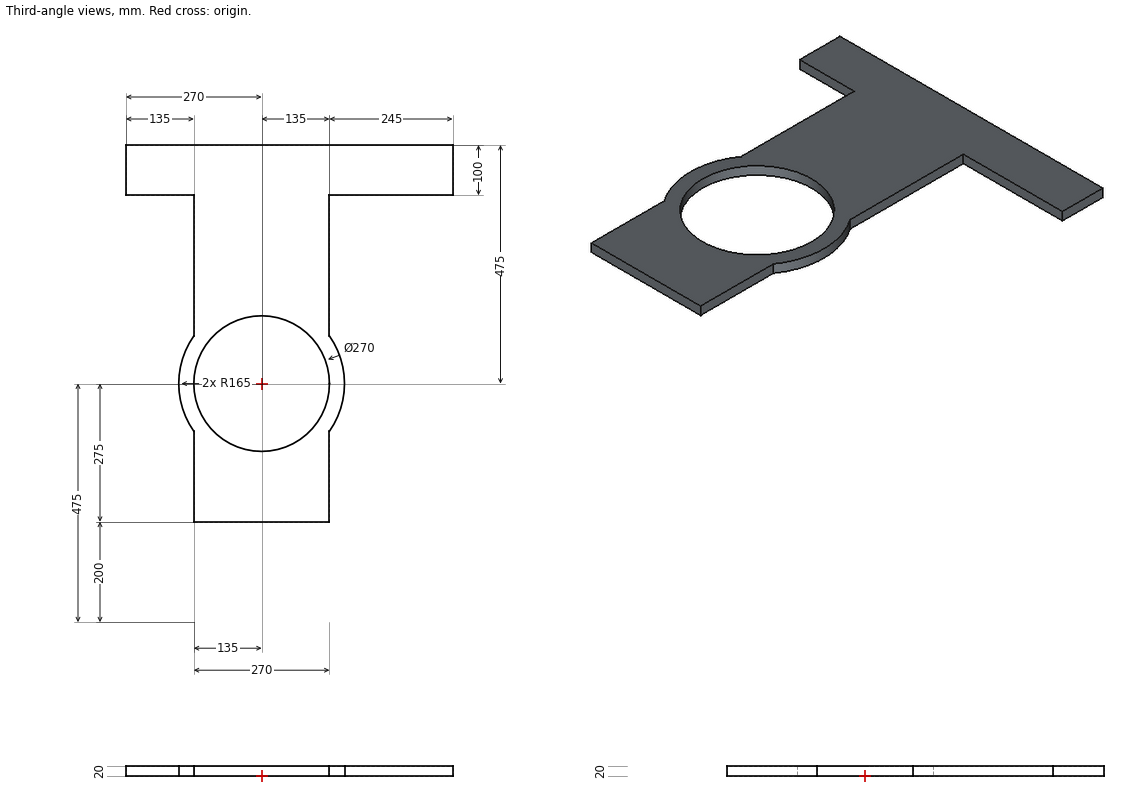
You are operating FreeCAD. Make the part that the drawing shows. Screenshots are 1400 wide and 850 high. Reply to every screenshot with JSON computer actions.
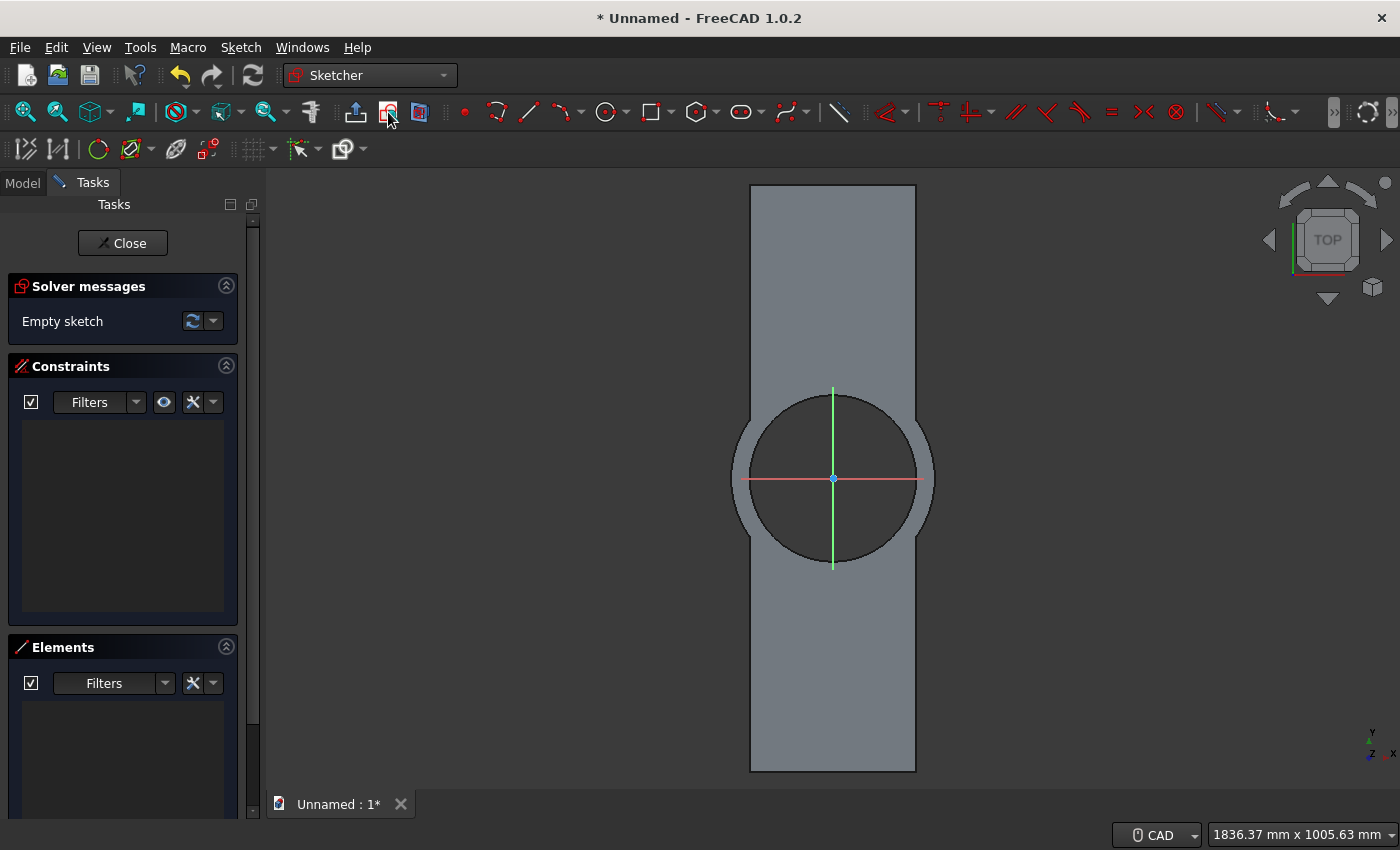
{"action": "scroll", "coordinate": [455, 196], "scroll_direction": "down", "scroll_amount": 1}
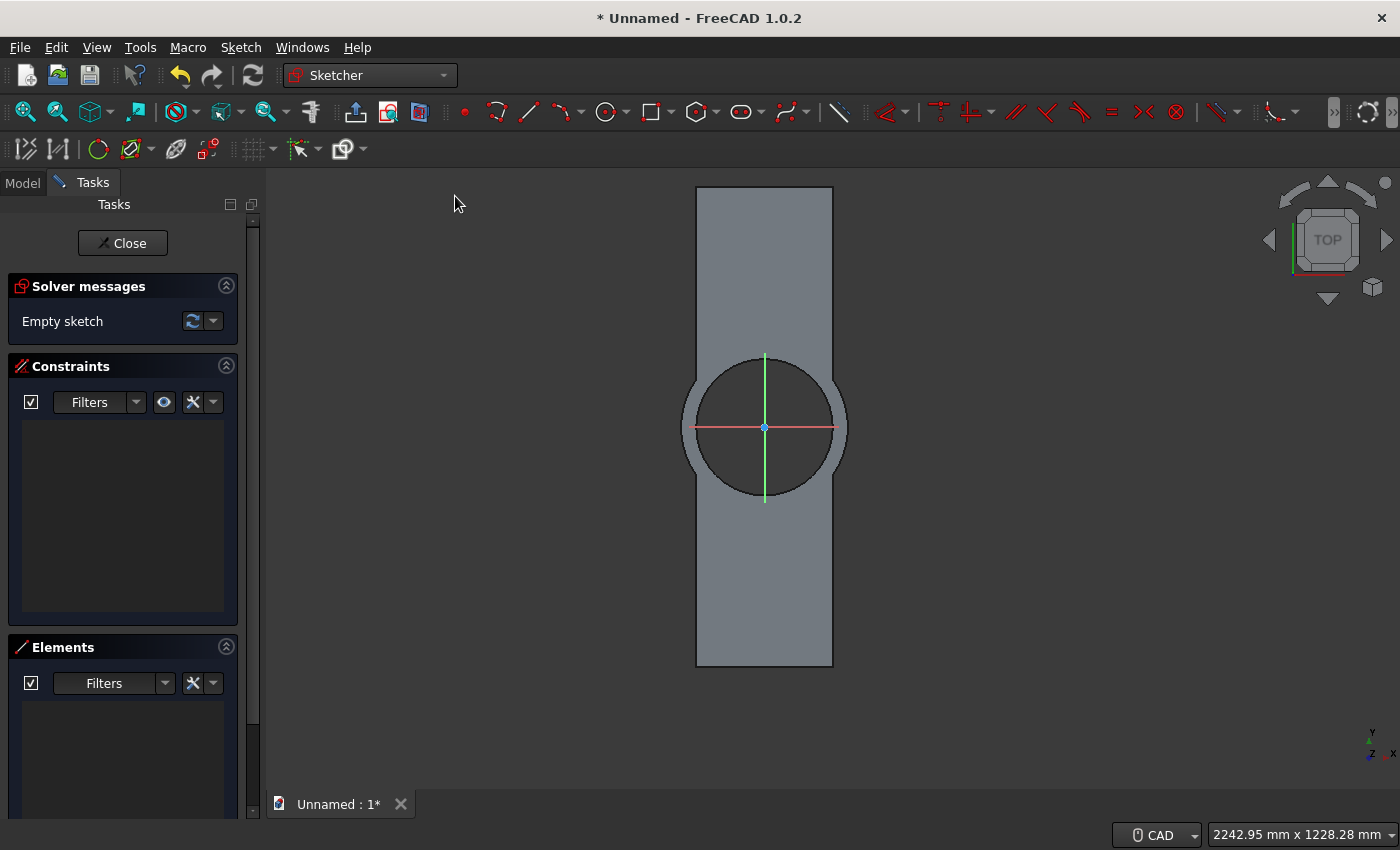
{"action": "scroll", "coordinate": [765, 631], "scroll_direction": "up", "scroll_amount": 3}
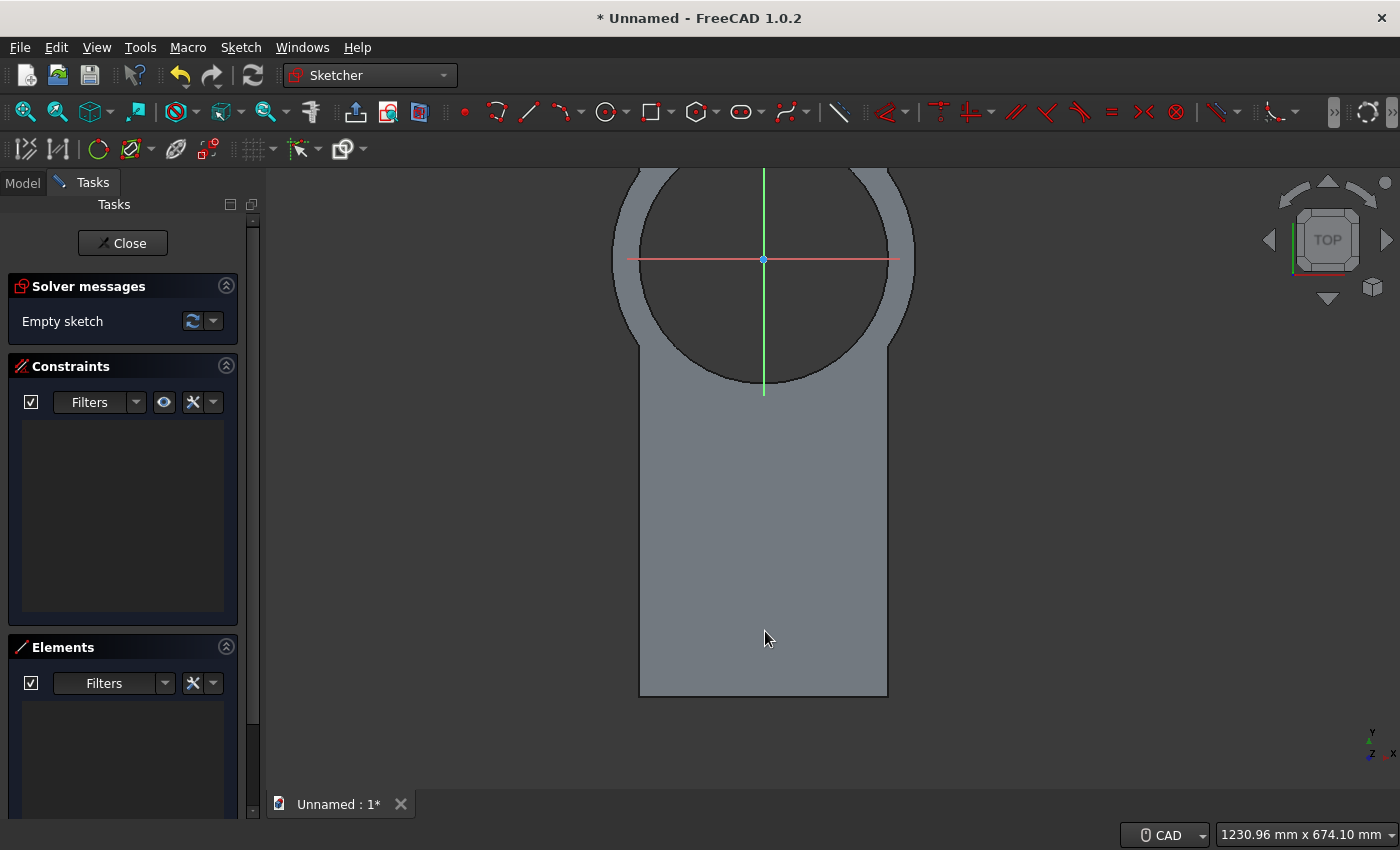
{"action": "left_click", "coordinate": [652, 112]}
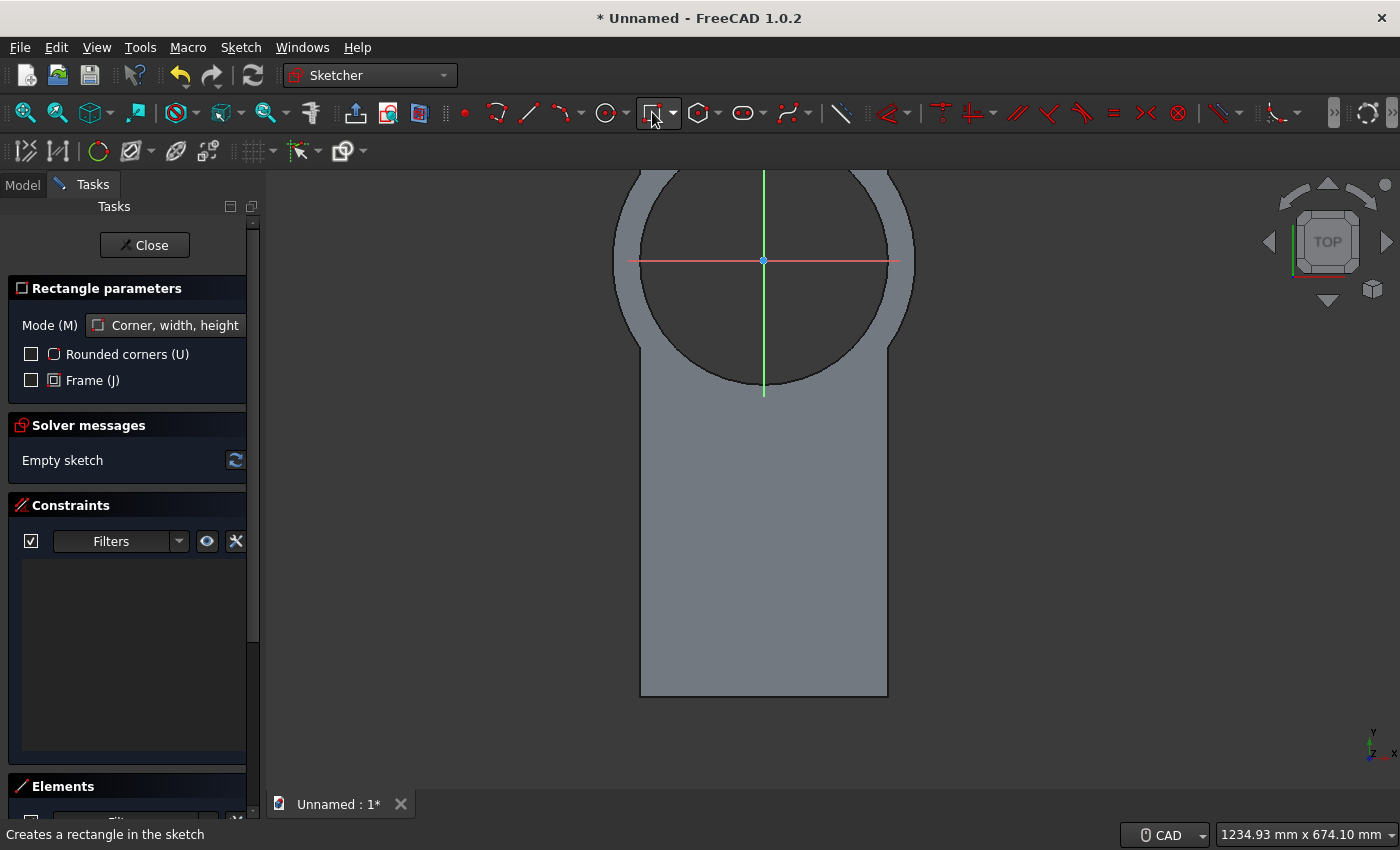
{"action": "left_click", "coordinate": [640, 513]}
{"action": "left_click", "coordinate": [888, 697]}
{"action": "key", "text": "Escape"}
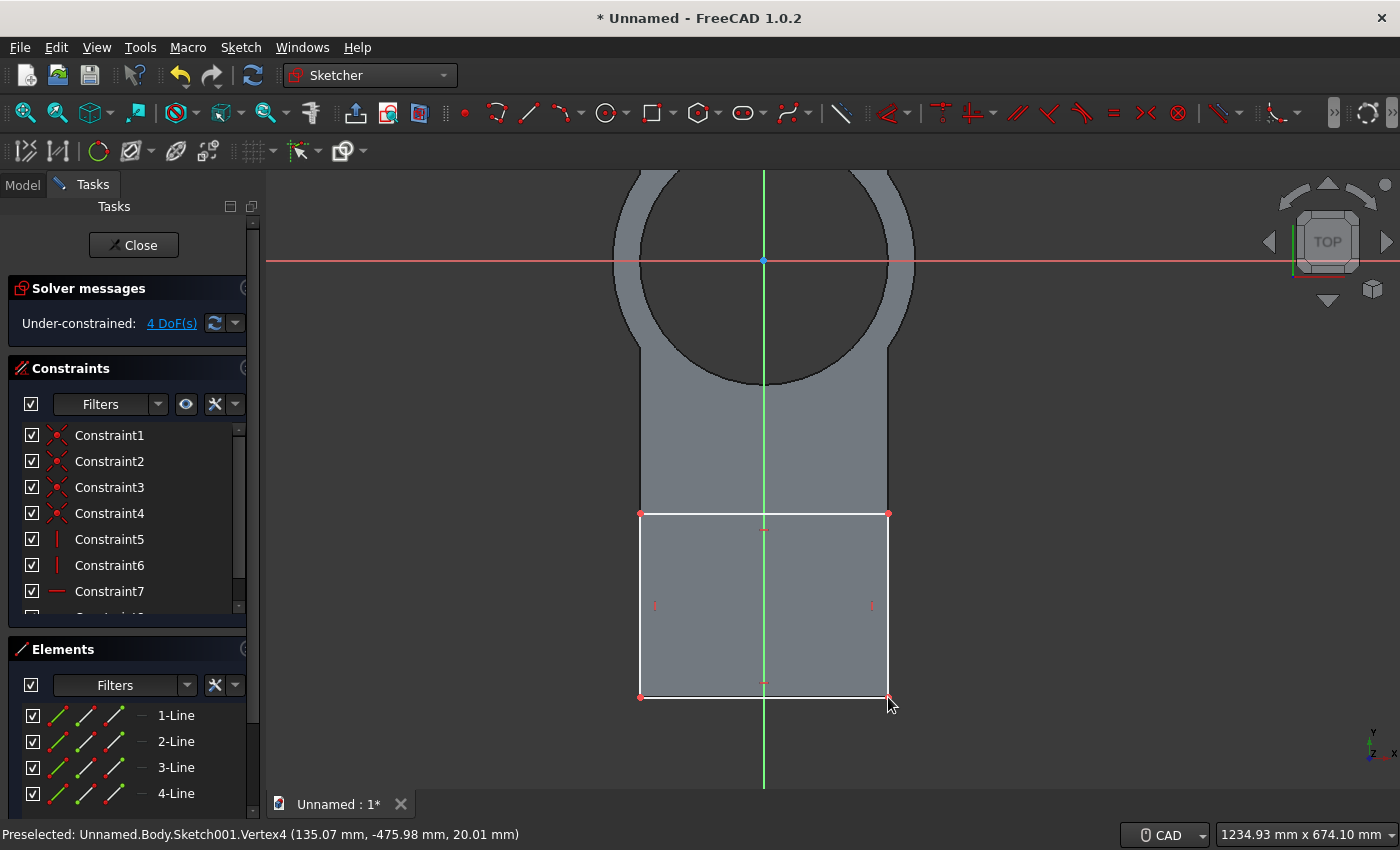
{"action": "left_click", "coordinate": [888, 114]}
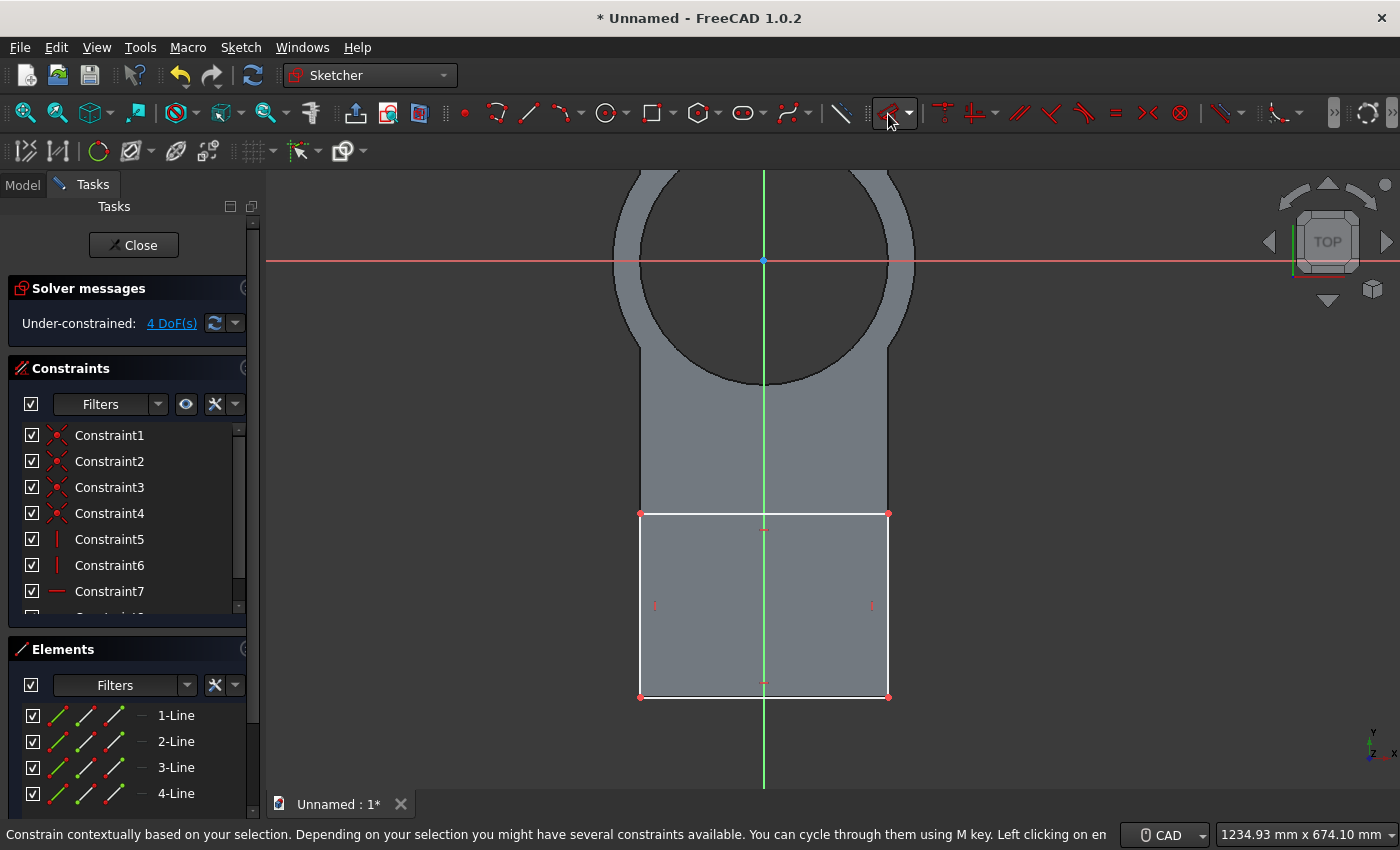
{"action": "left_click", "coordinate": [640, 569]}
{"action": "left_click", "coordinate": [606, 606]}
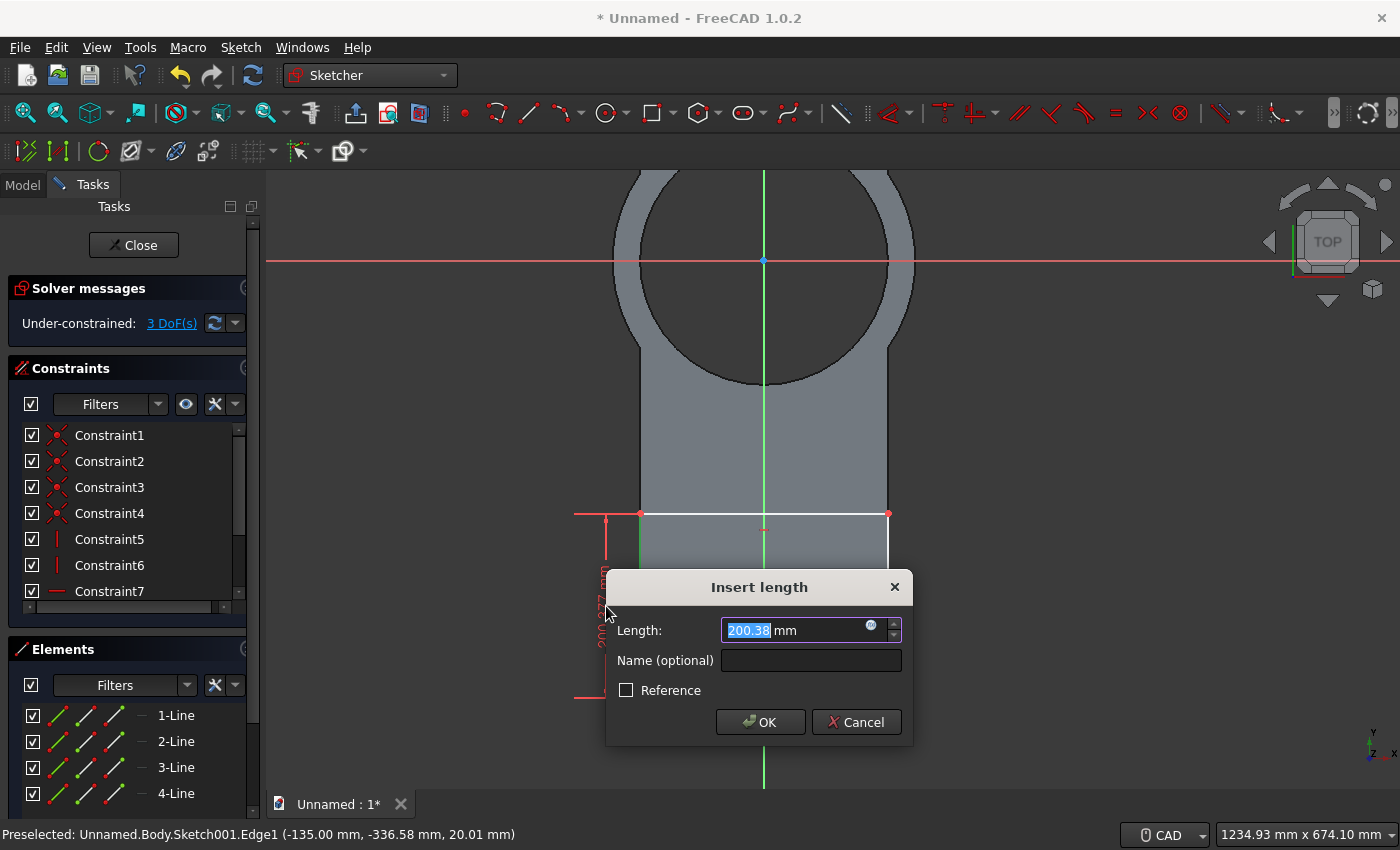
{"action": "type", "text": "200"}
{"action": "key", "text": "Return"}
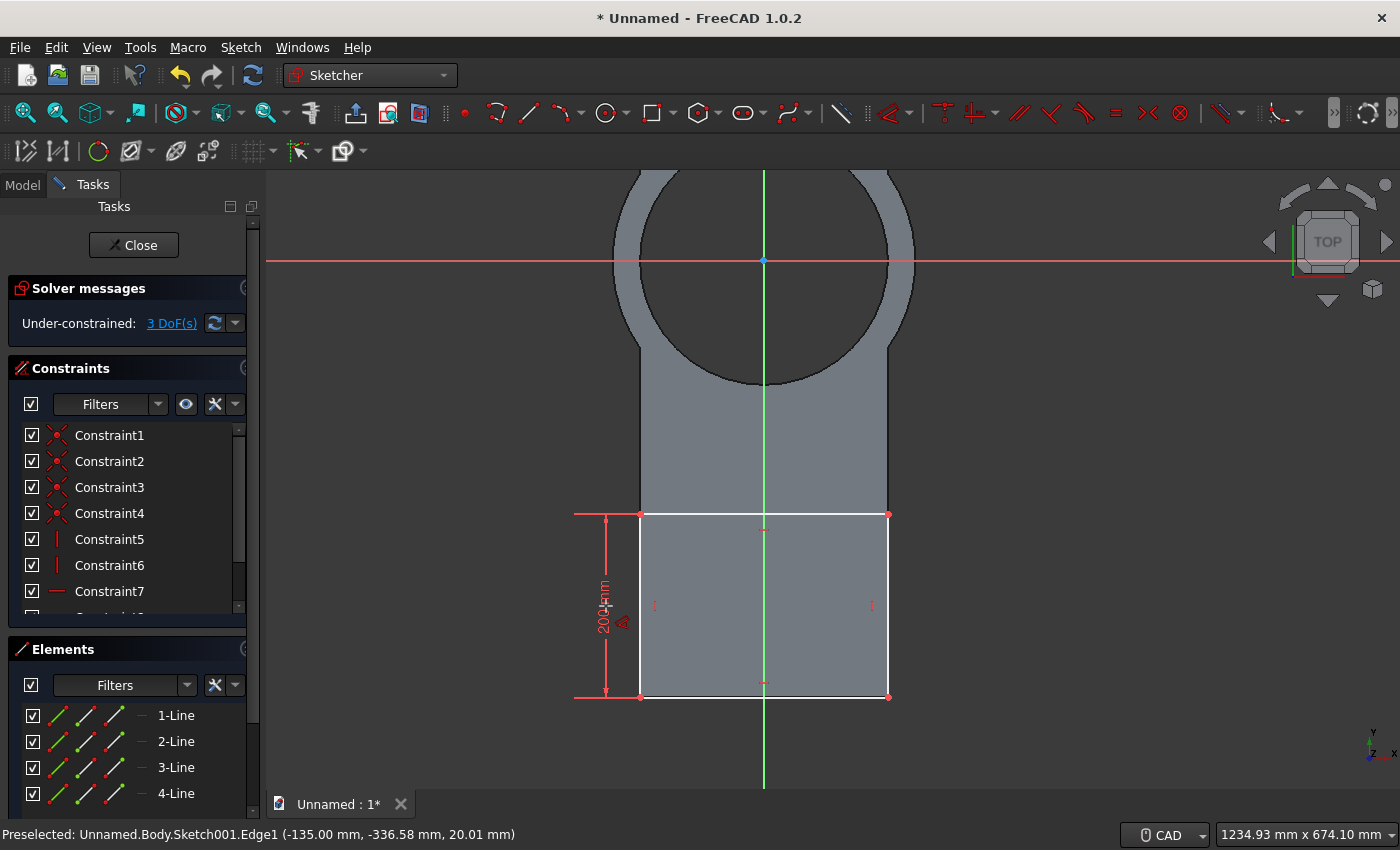
{"action": "left_click", "coordinate": [714, 698]}
{"action": "left_click", "coordinate": [707, 732]}